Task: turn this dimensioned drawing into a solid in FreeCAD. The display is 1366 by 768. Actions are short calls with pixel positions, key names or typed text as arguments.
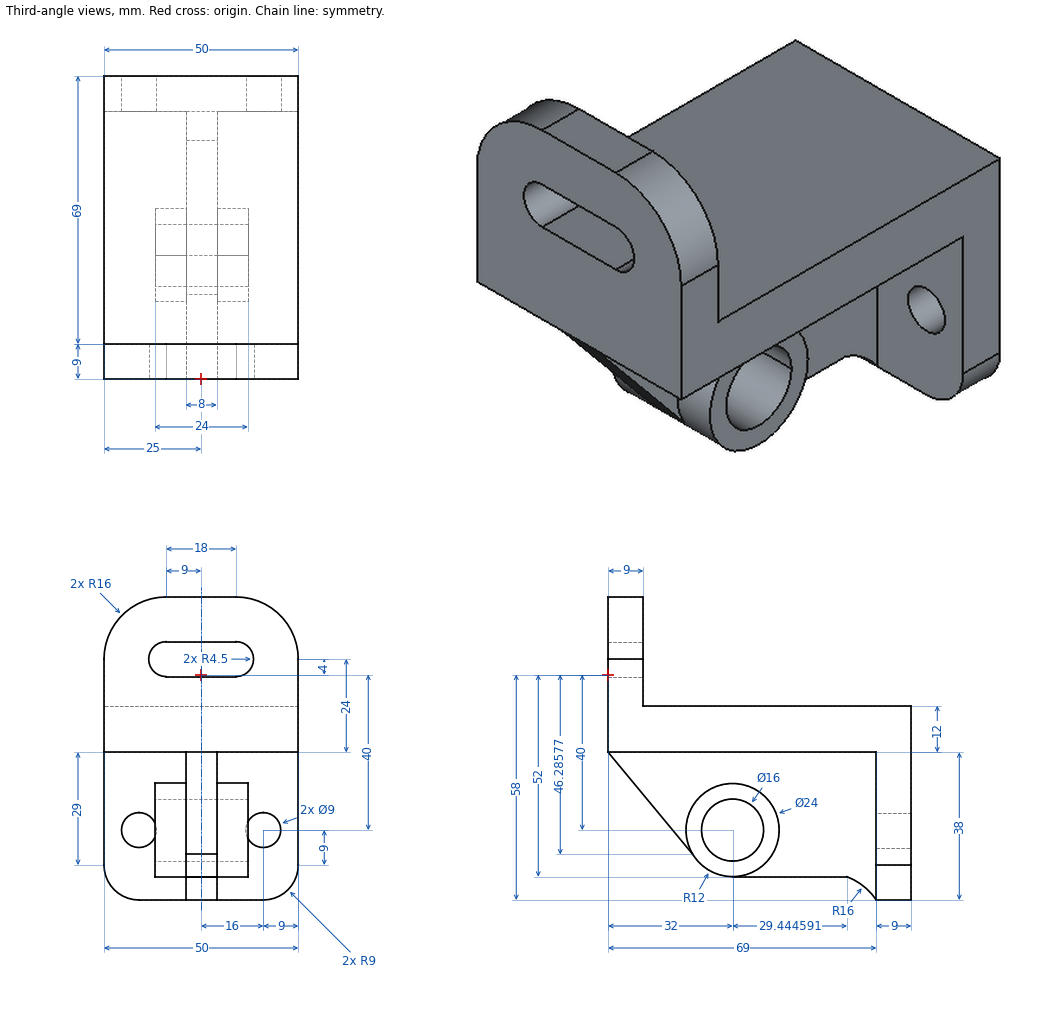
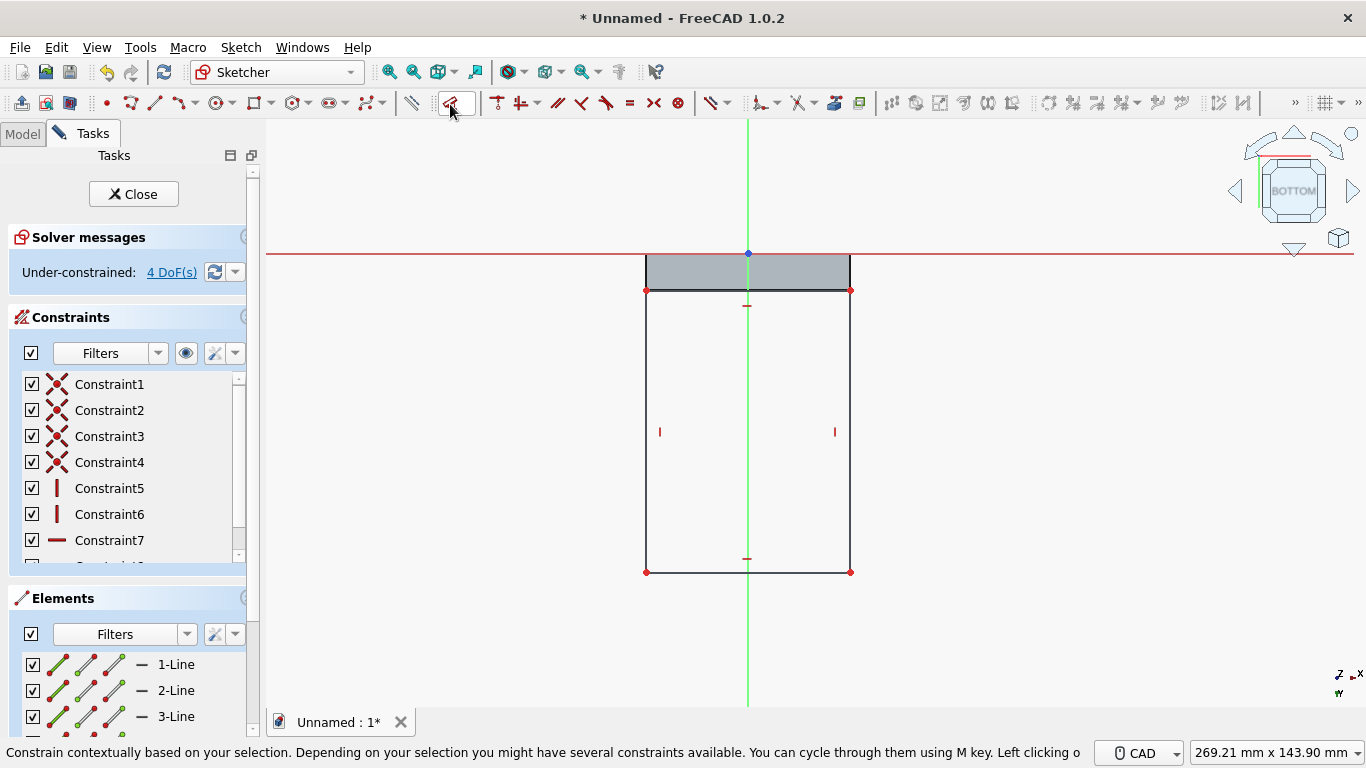
click(646, 376)
click(612, 432)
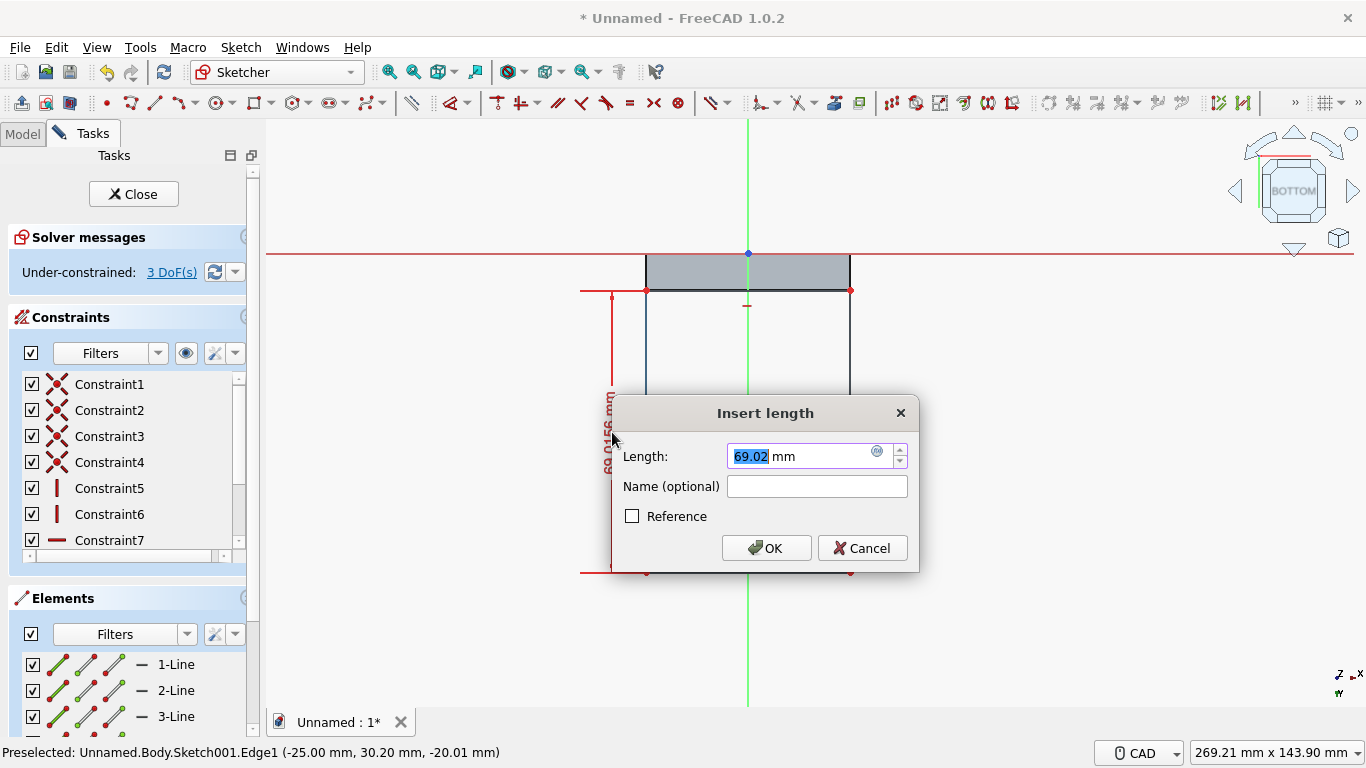
text(69)
key(Return)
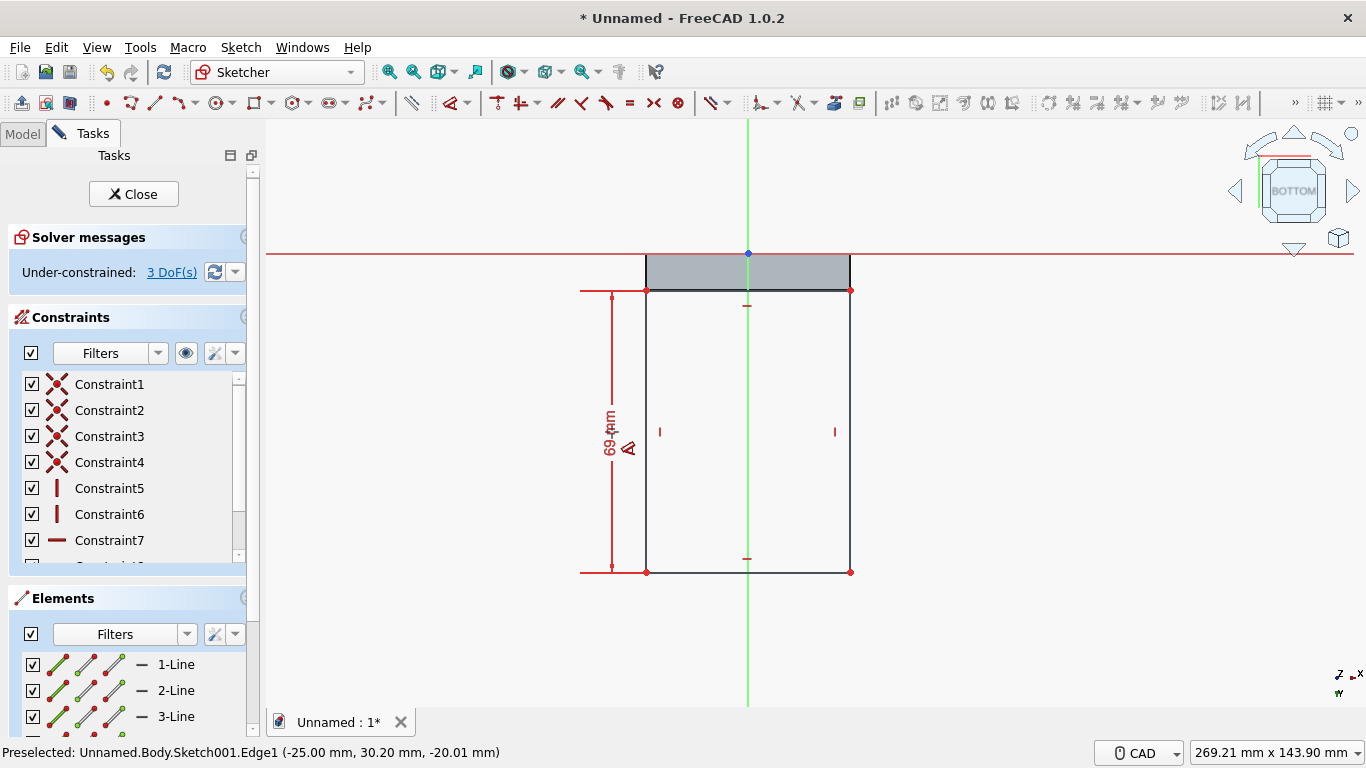
click(707, 573)
click(701, 607)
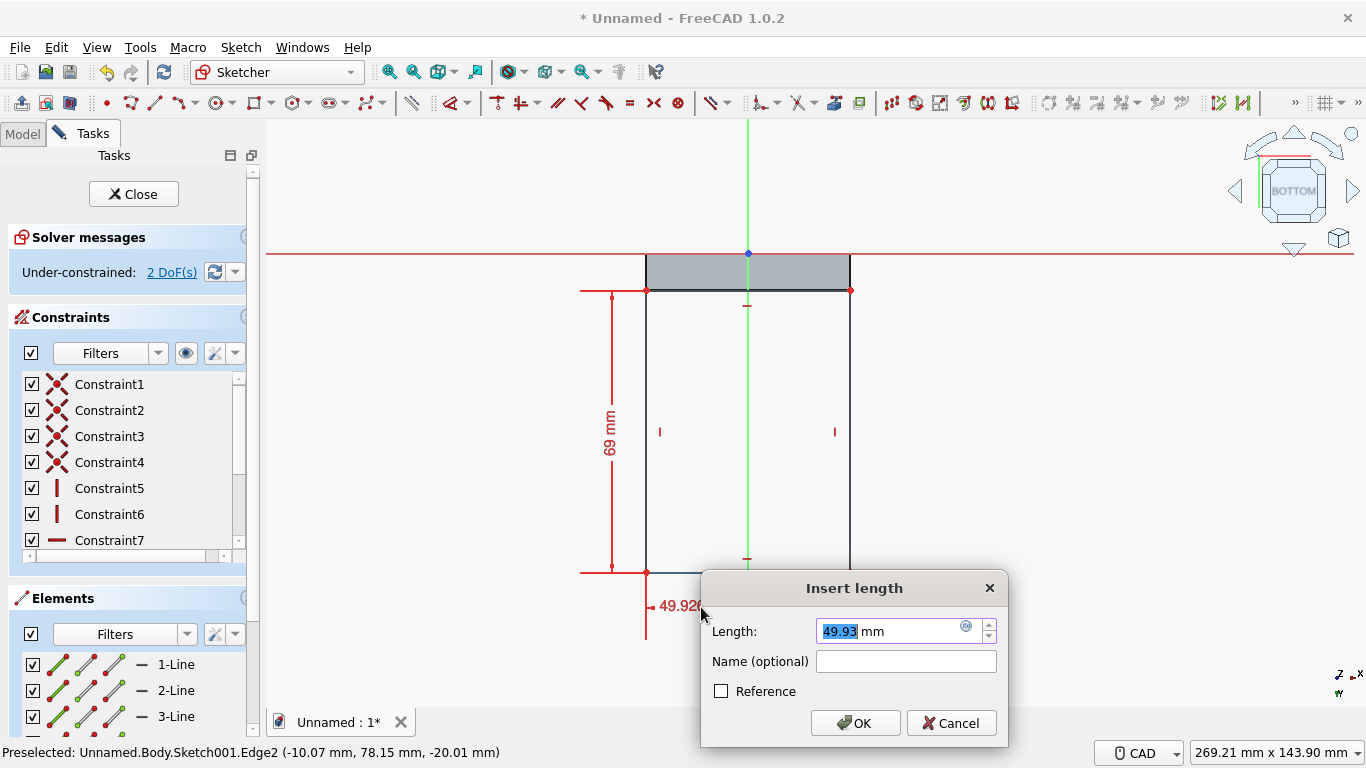
text(50)
key(Return)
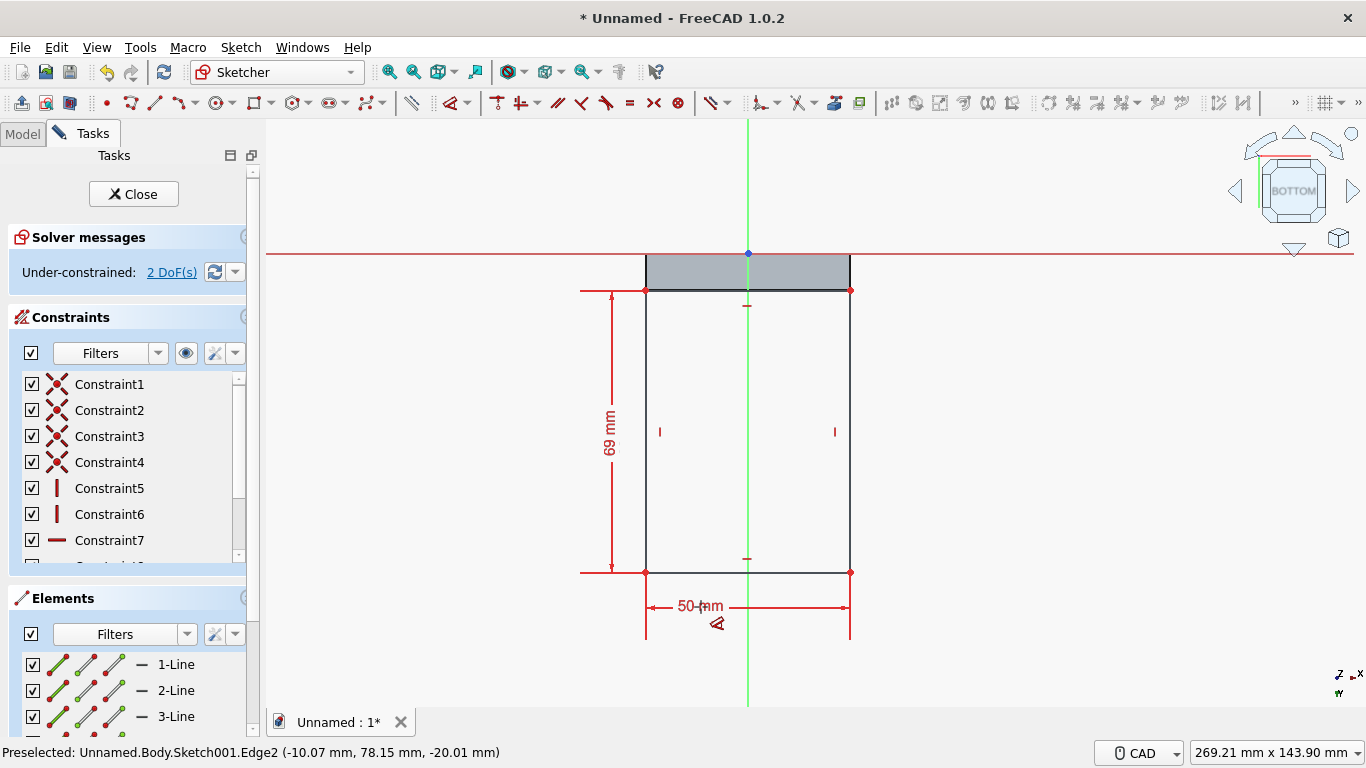
click(646, 291)
click(612, 272)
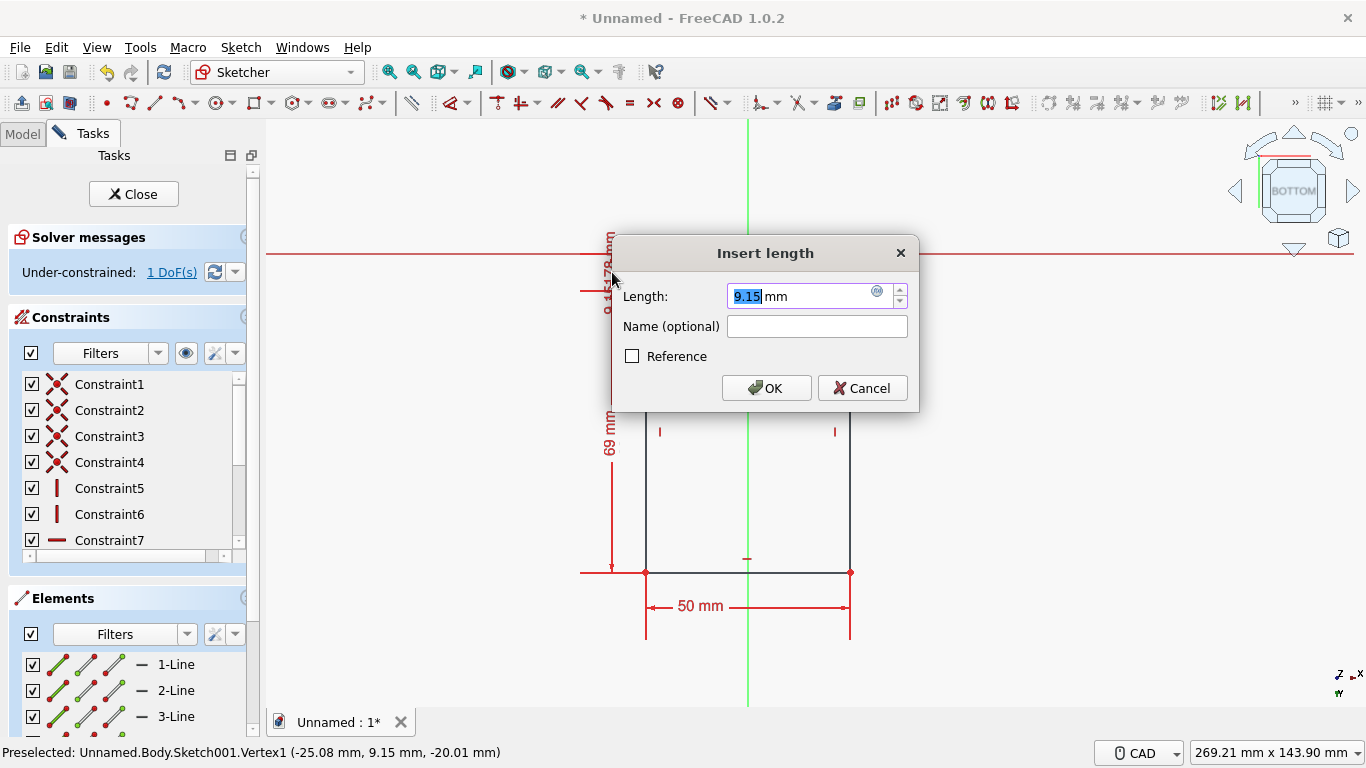
text(9)
key(Return)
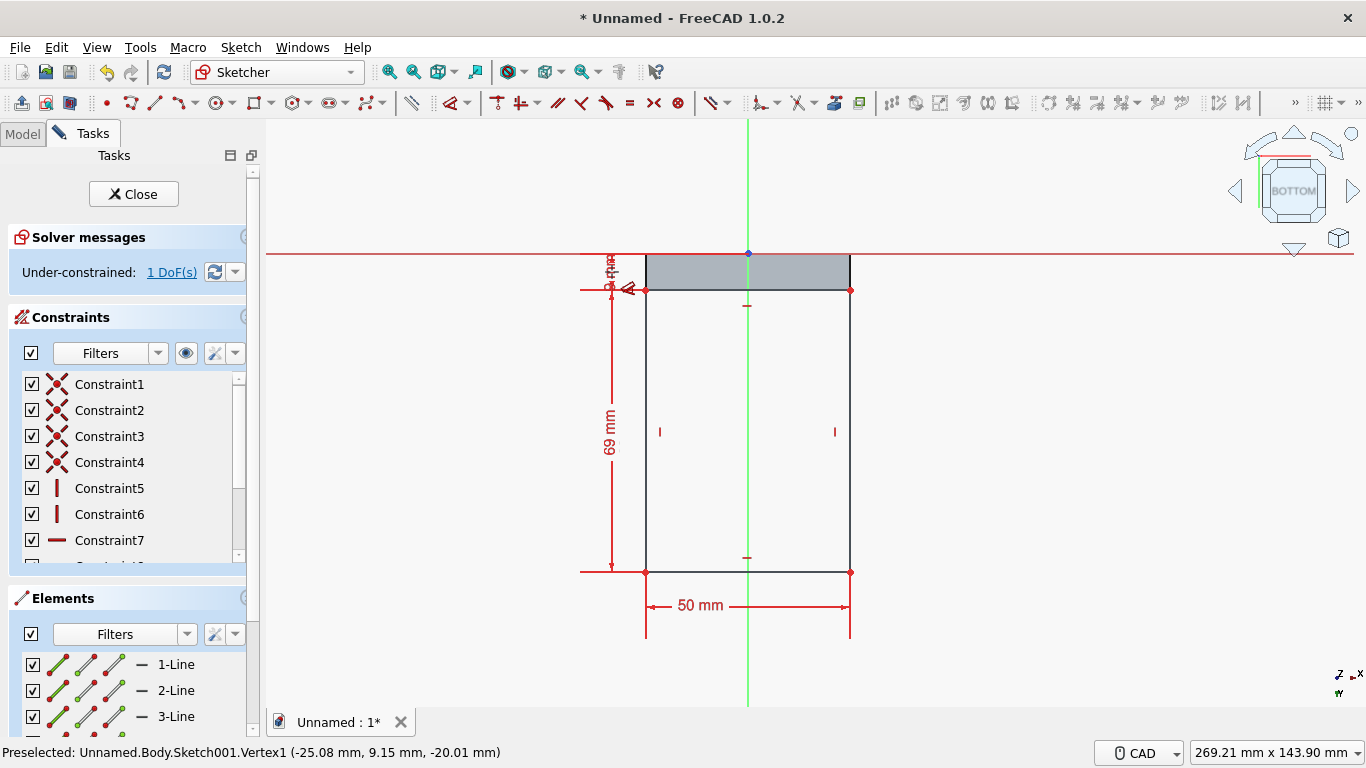
click(646, 290)
click(697, 220)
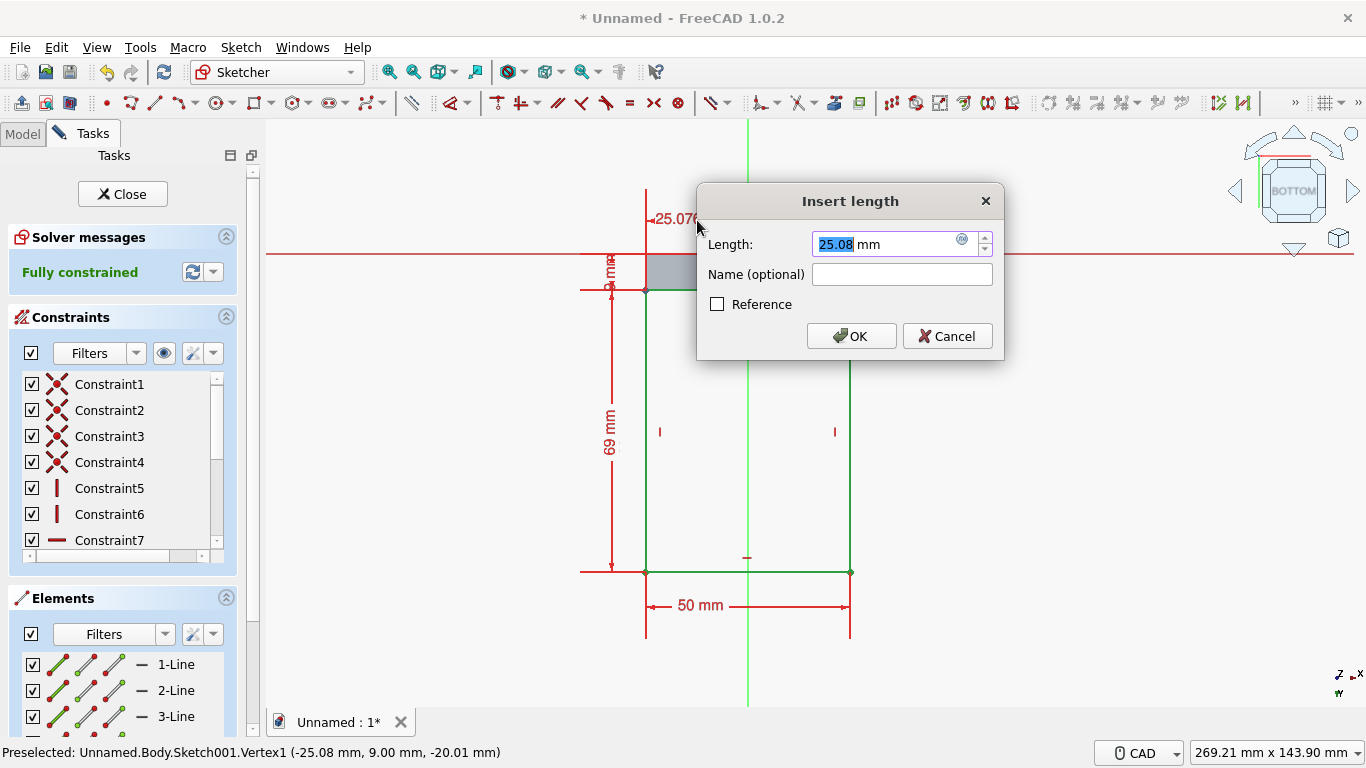
text(25)
key(Return)
key(Escape)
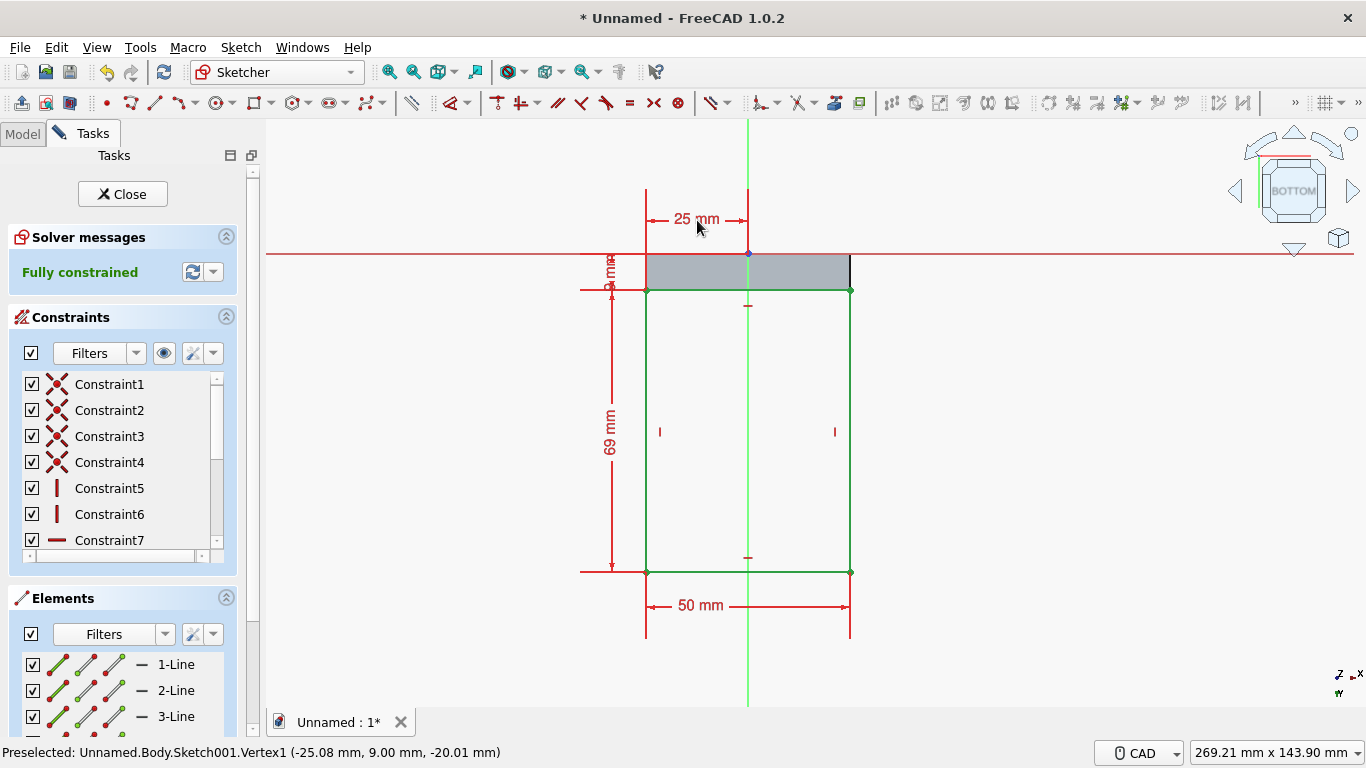
click(123, 194)